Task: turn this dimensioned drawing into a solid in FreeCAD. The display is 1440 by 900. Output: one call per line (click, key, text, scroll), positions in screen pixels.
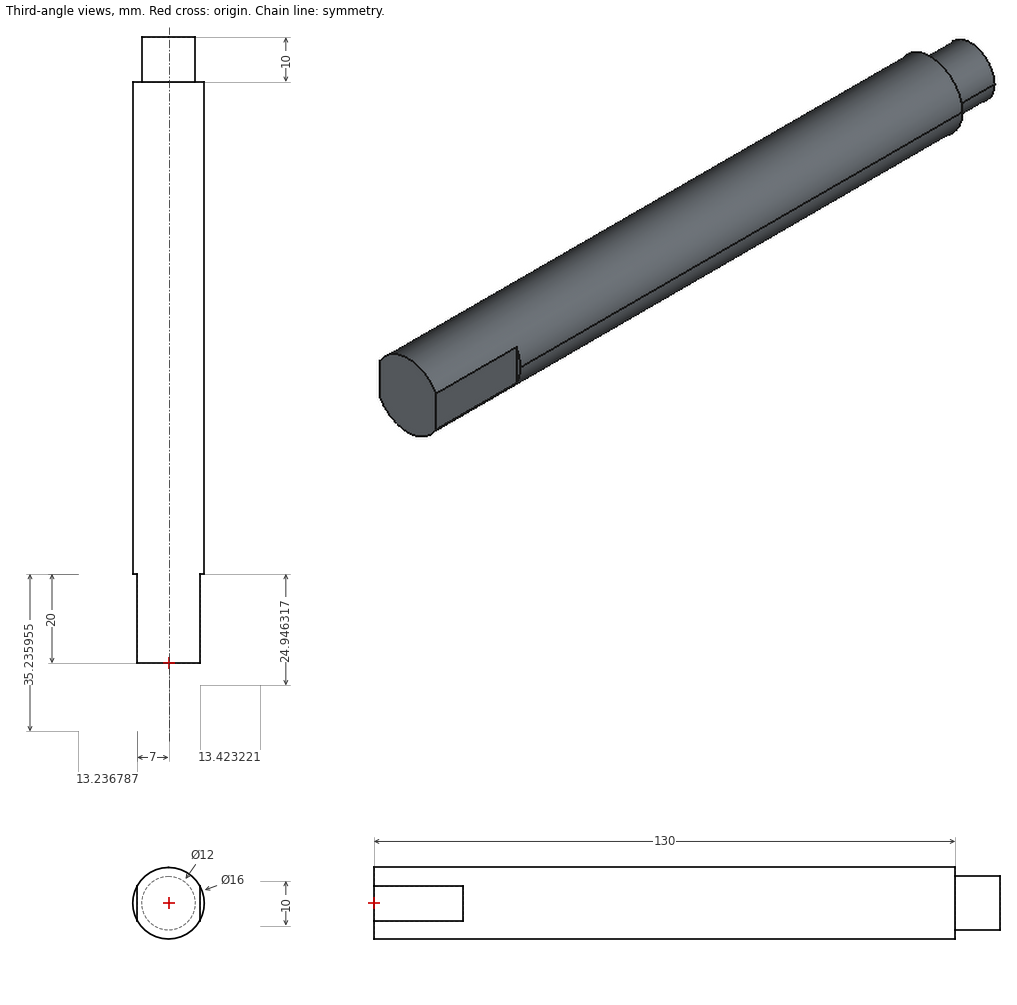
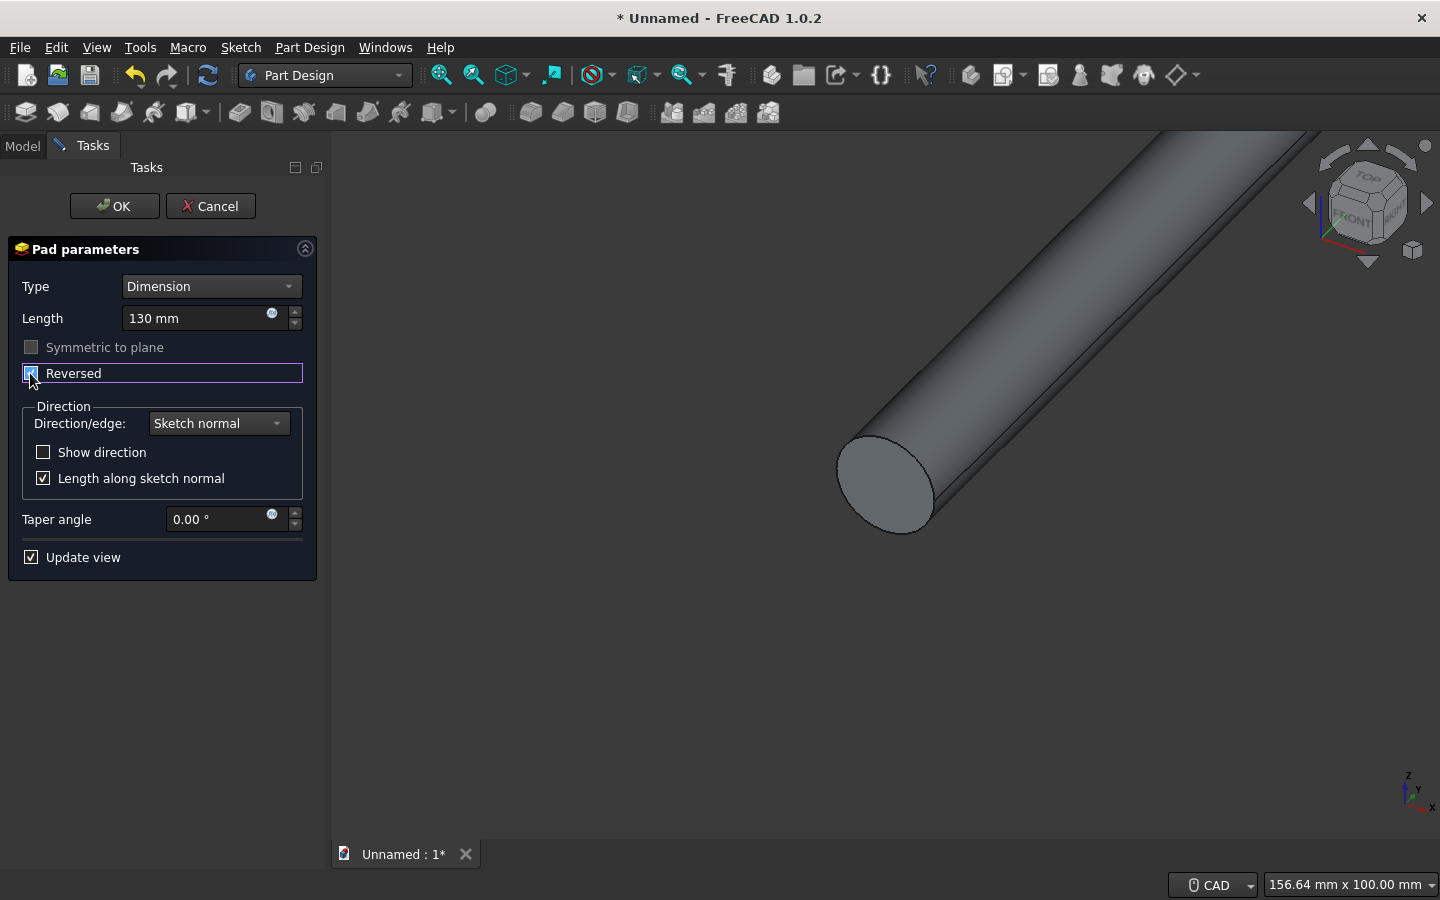
click(115, 206)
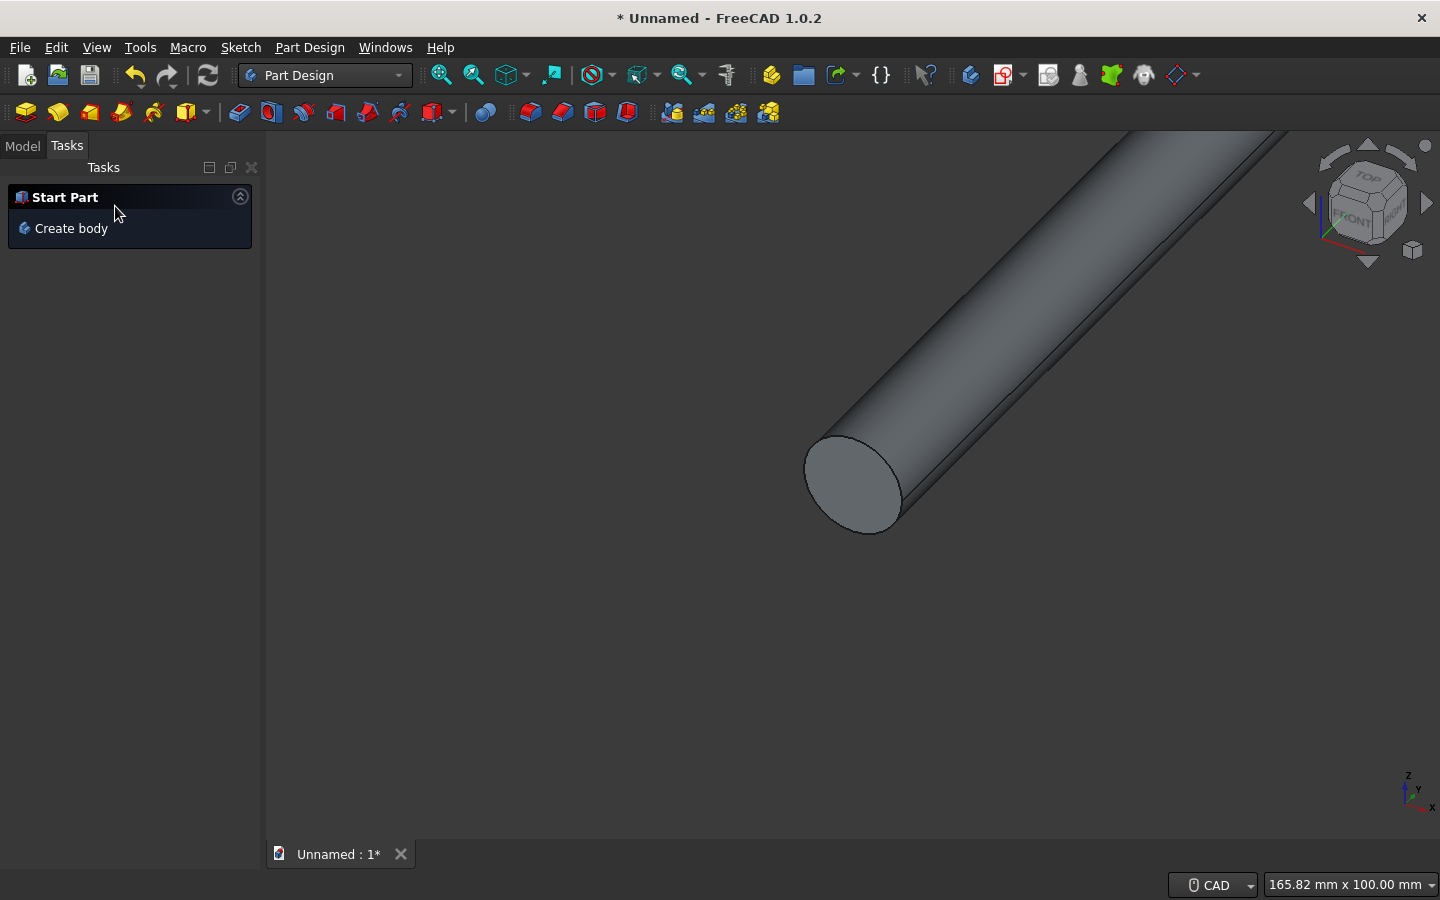
click(442, 76)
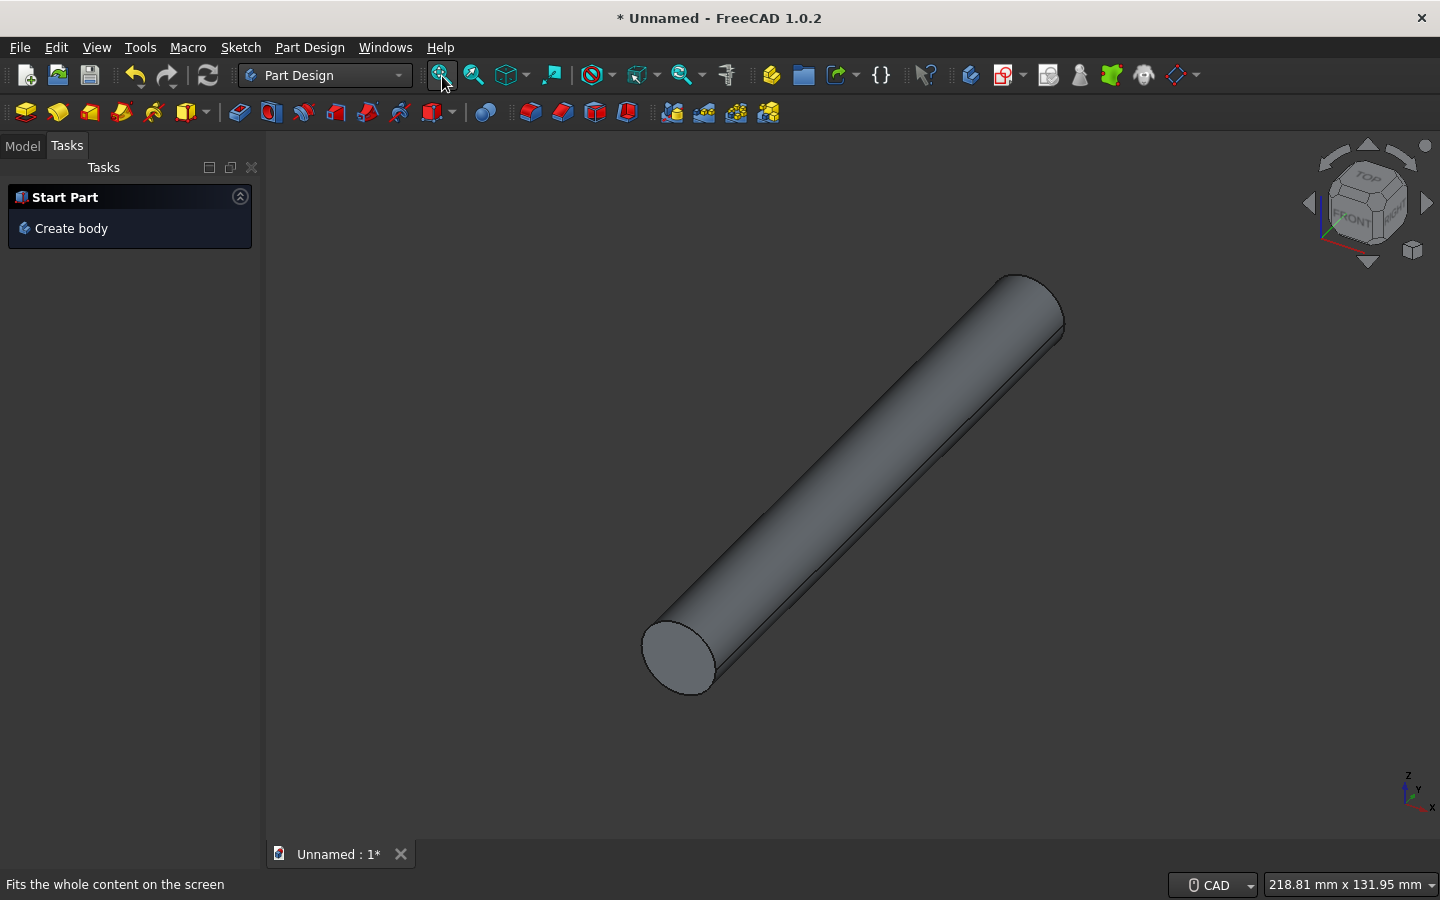
key(4)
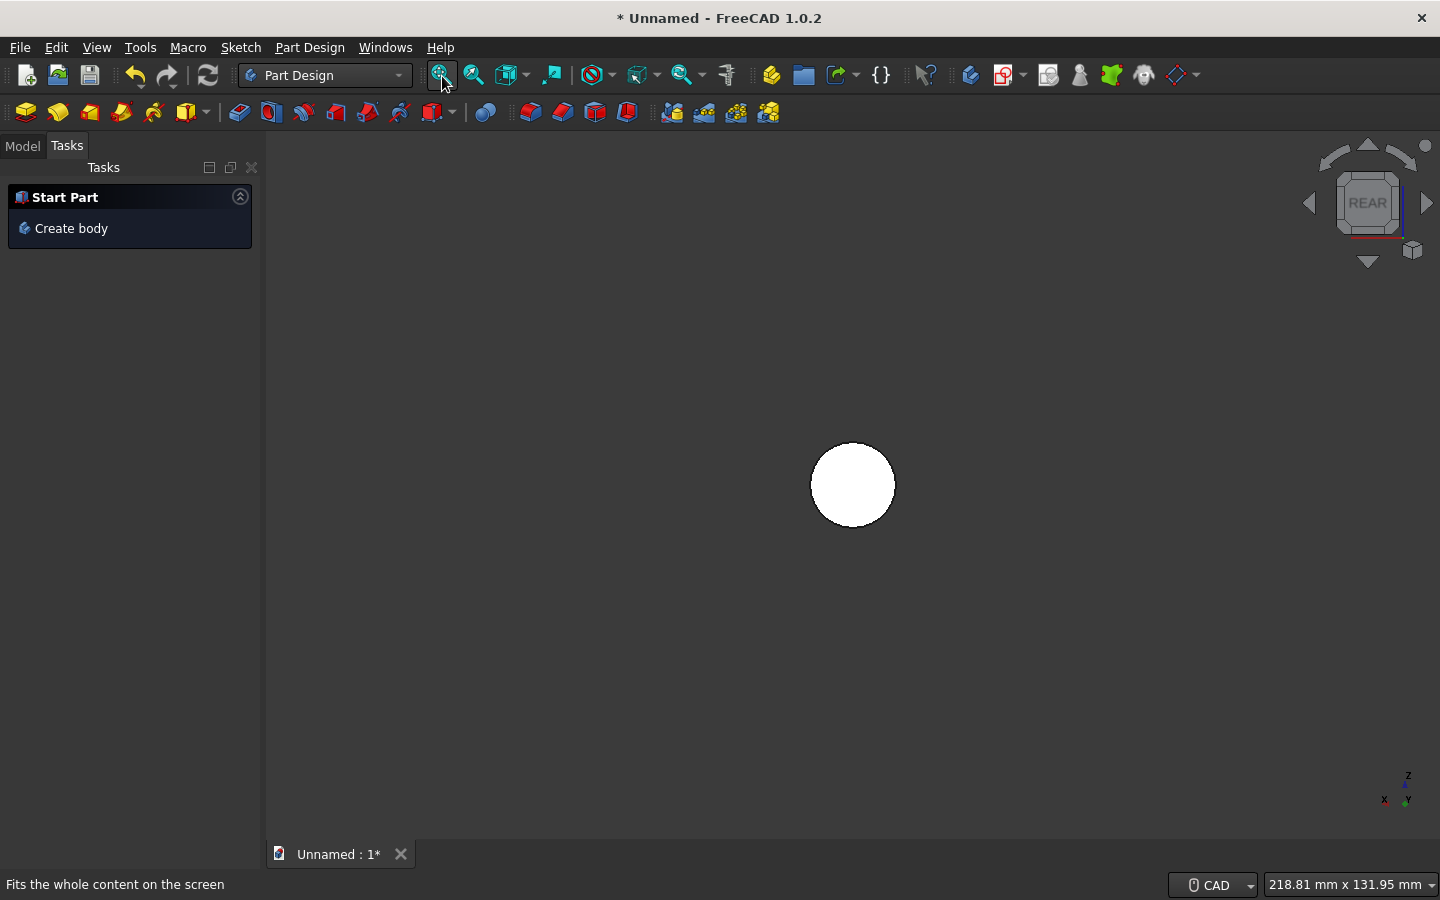
key(v)
key(f)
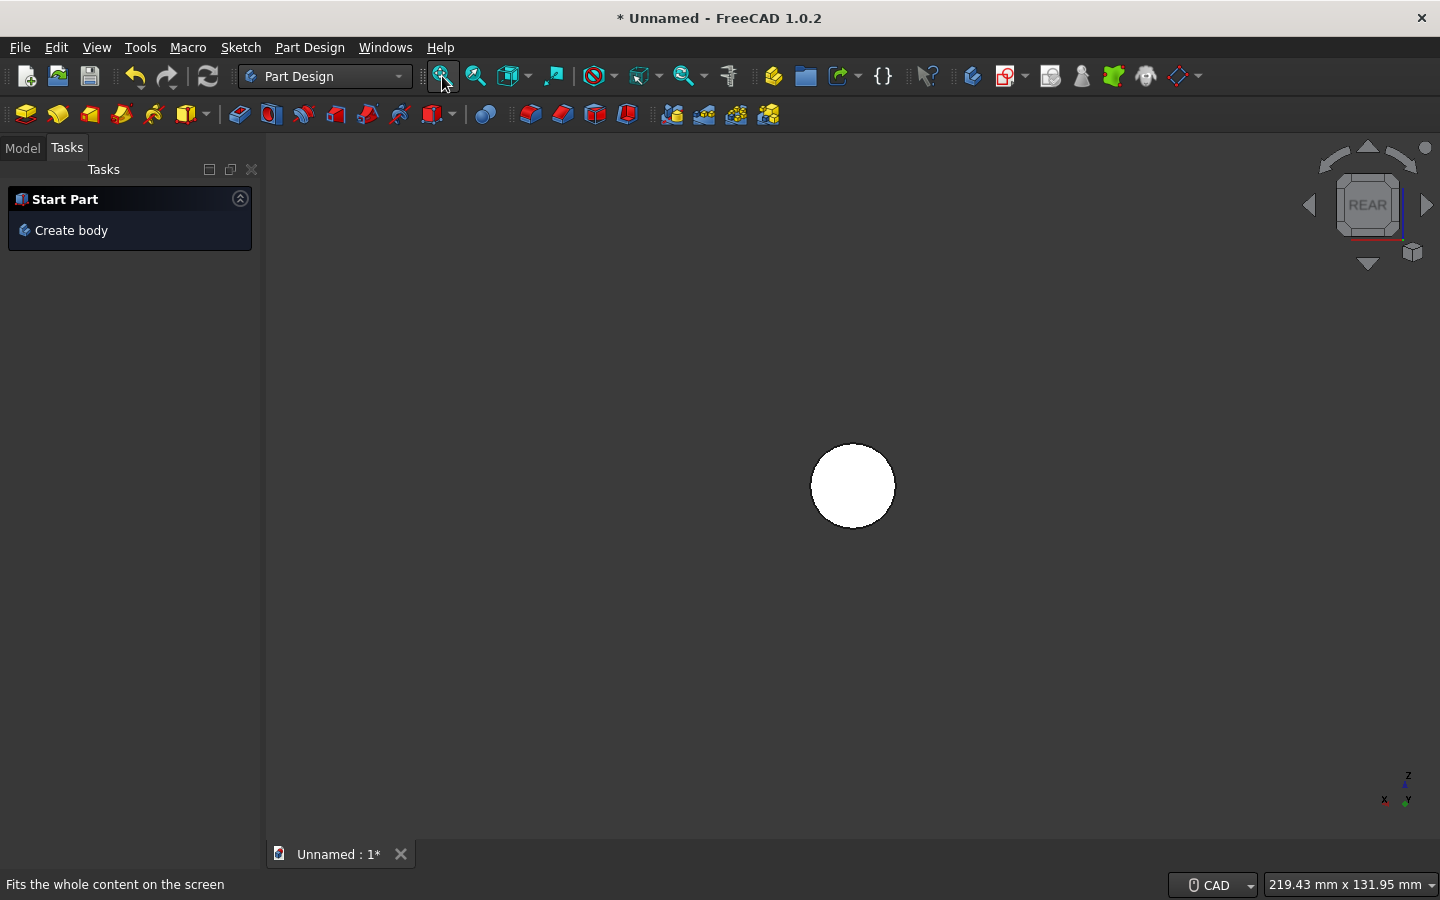
click(853, 485)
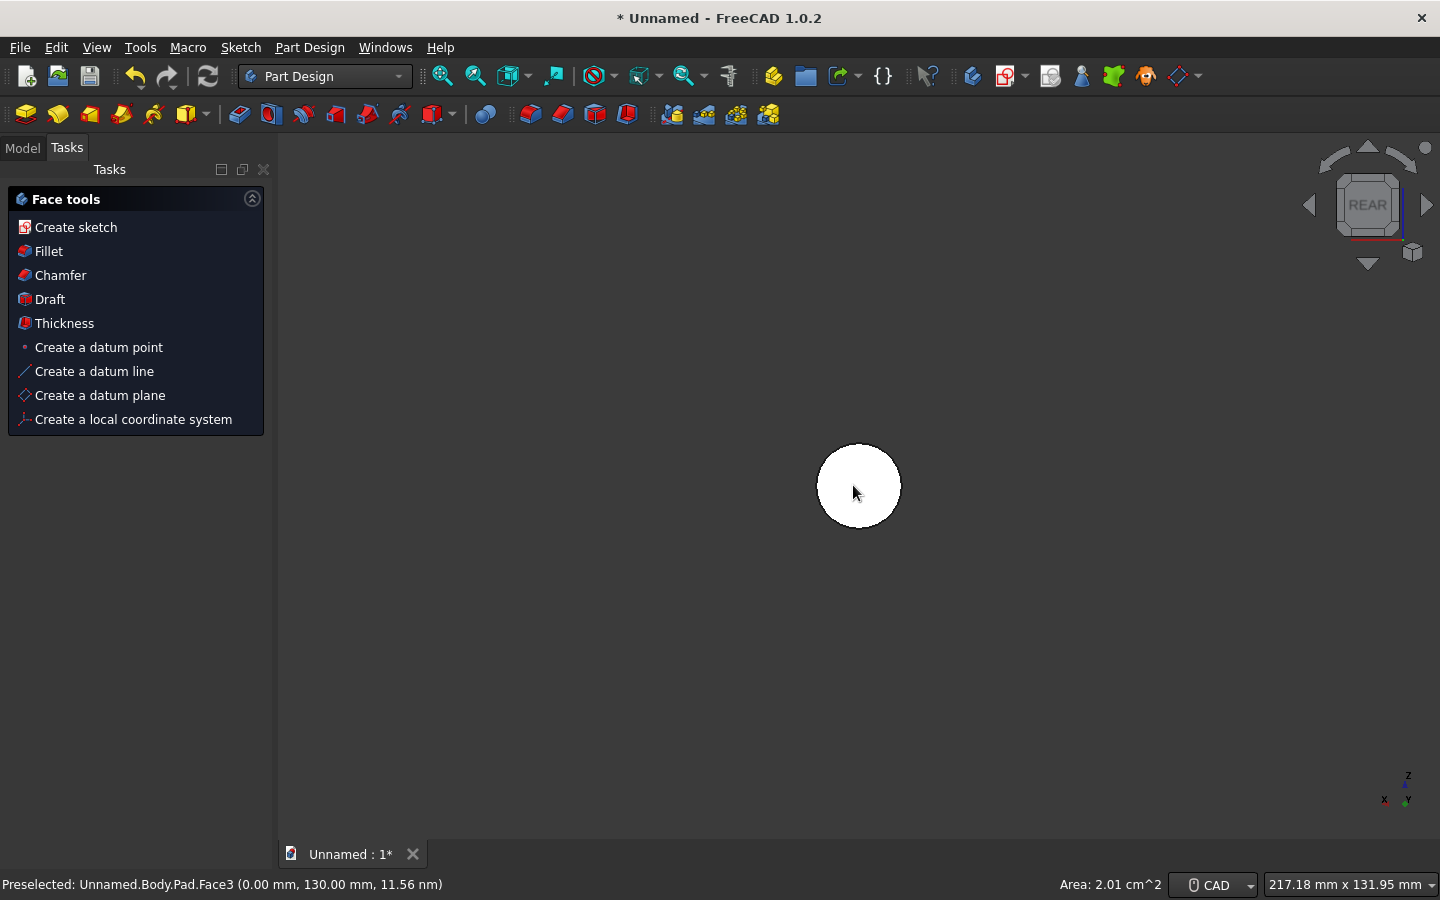
click(1006, 76)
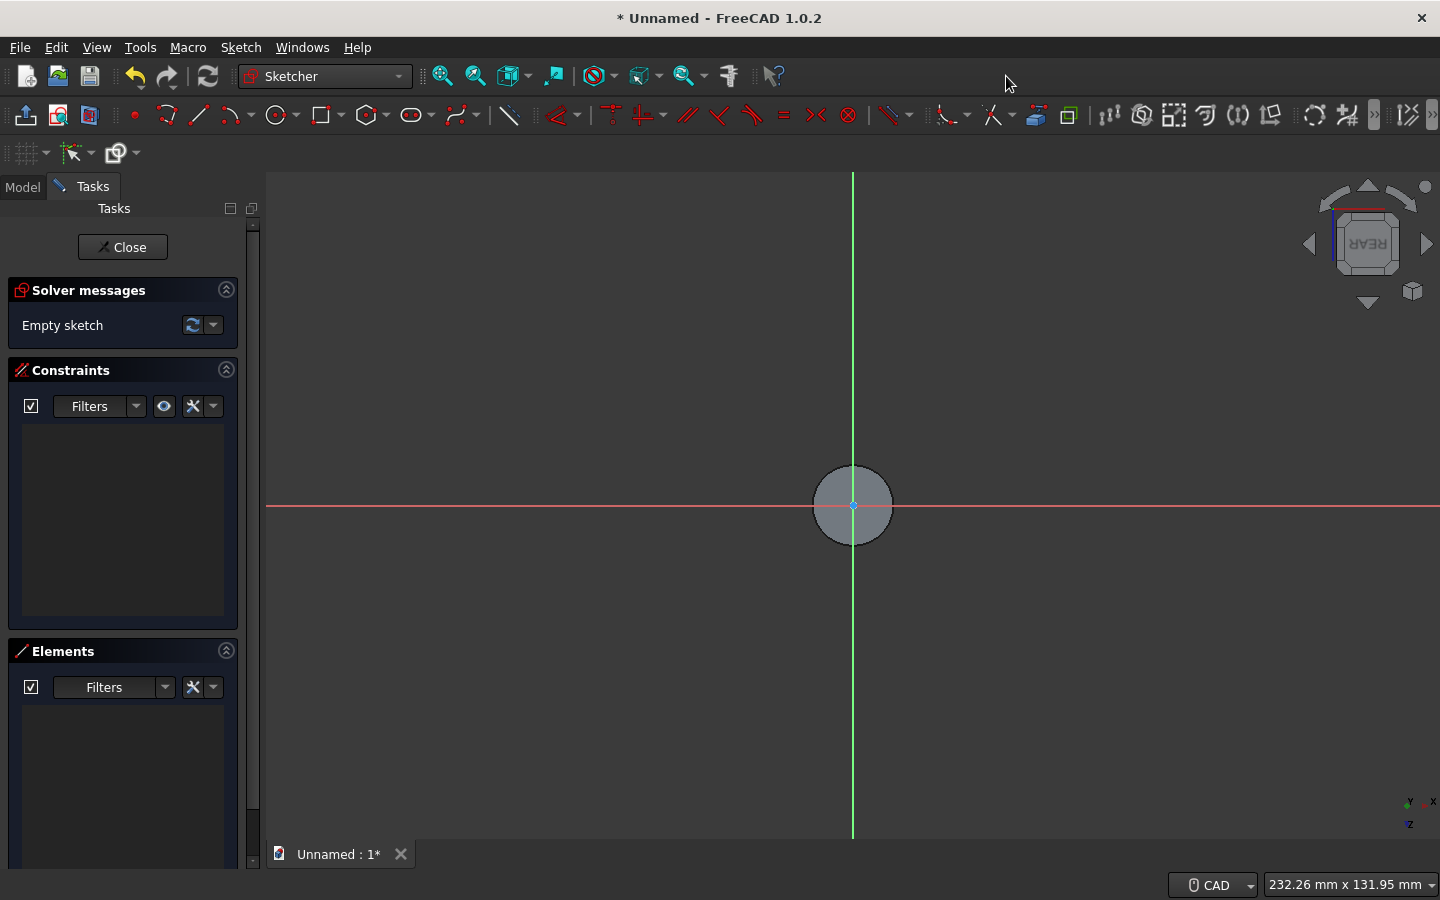
scroll(864, 505, up, 10)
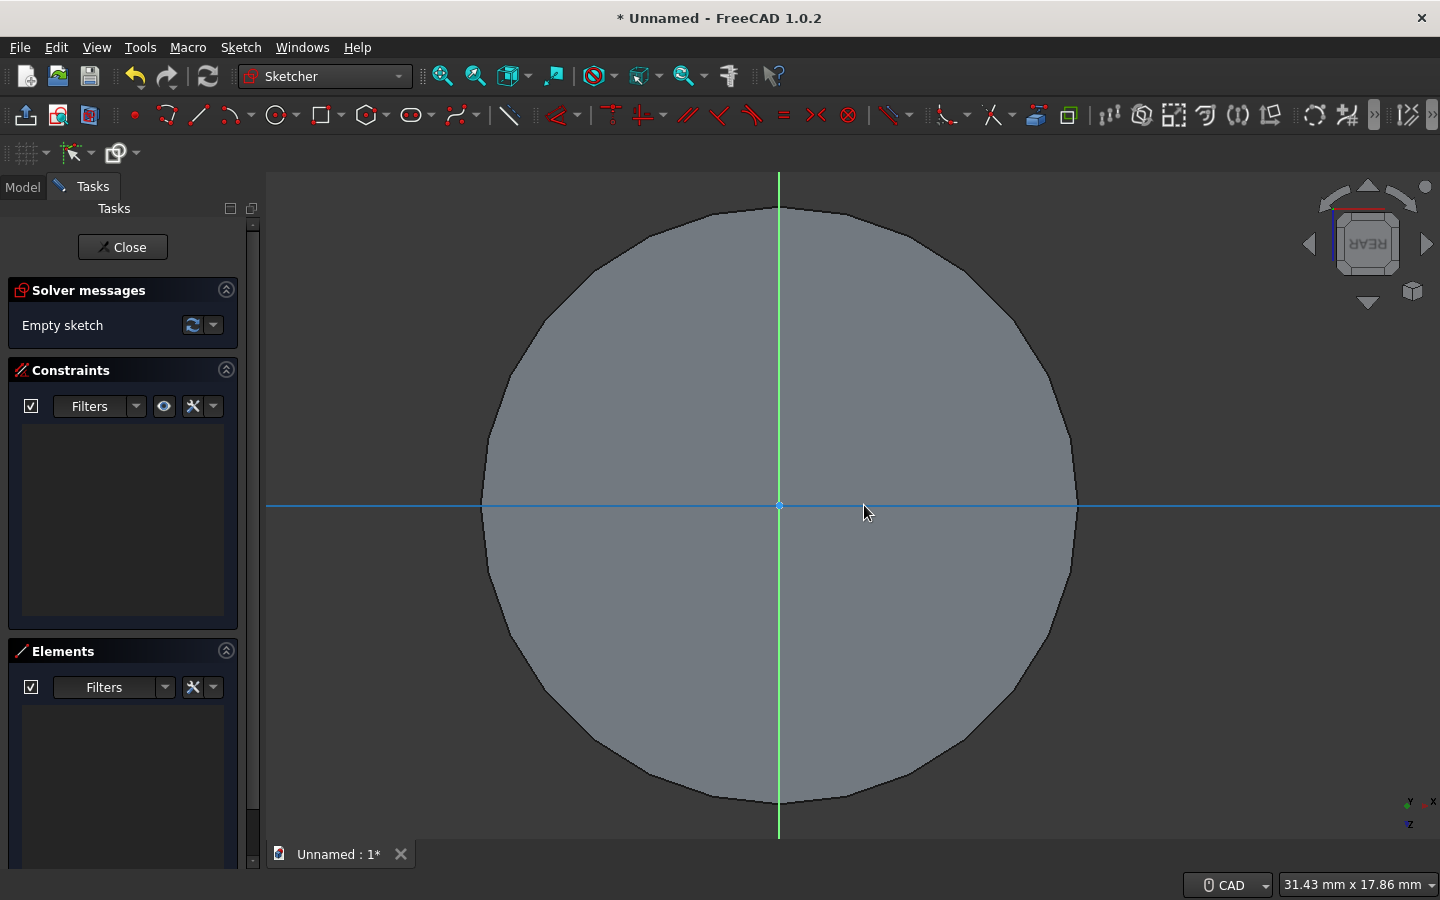
key(g)
key(c)